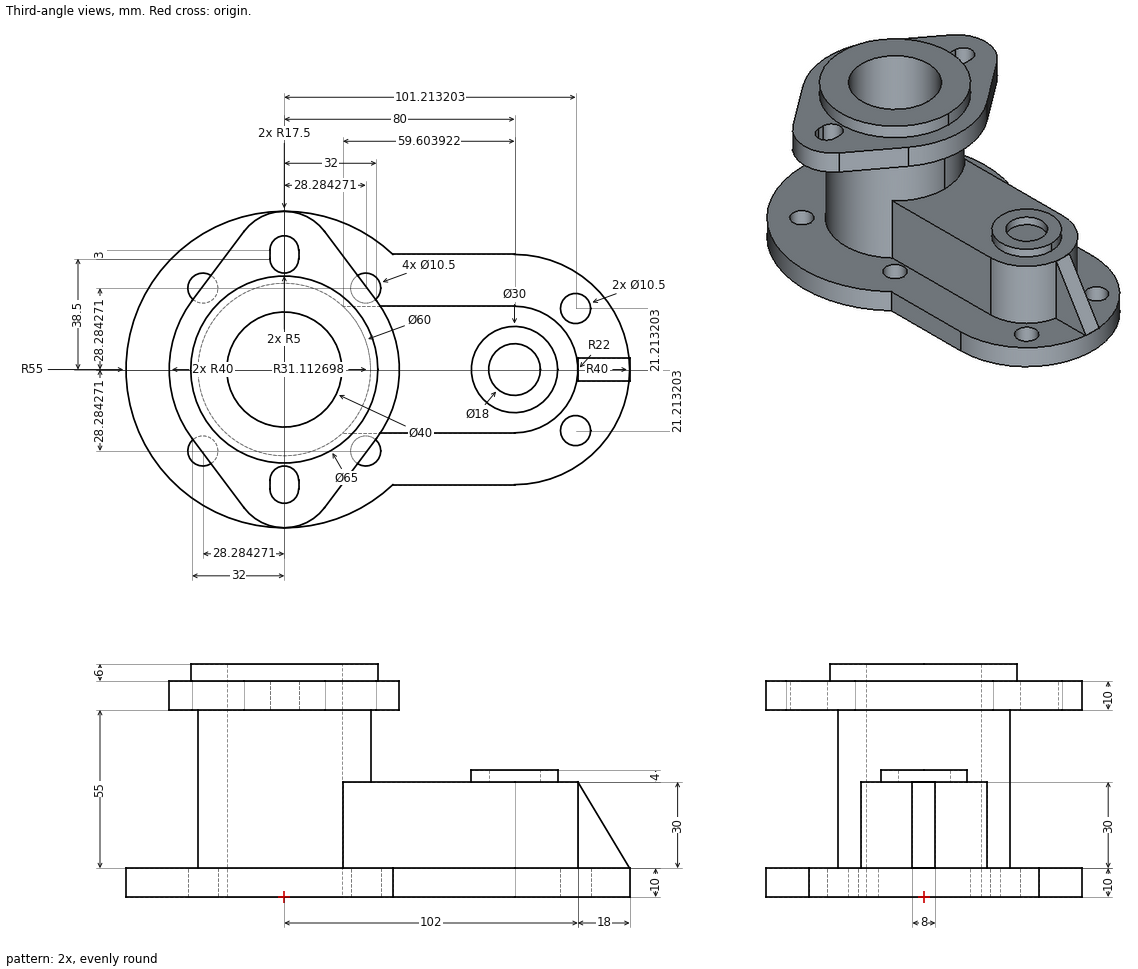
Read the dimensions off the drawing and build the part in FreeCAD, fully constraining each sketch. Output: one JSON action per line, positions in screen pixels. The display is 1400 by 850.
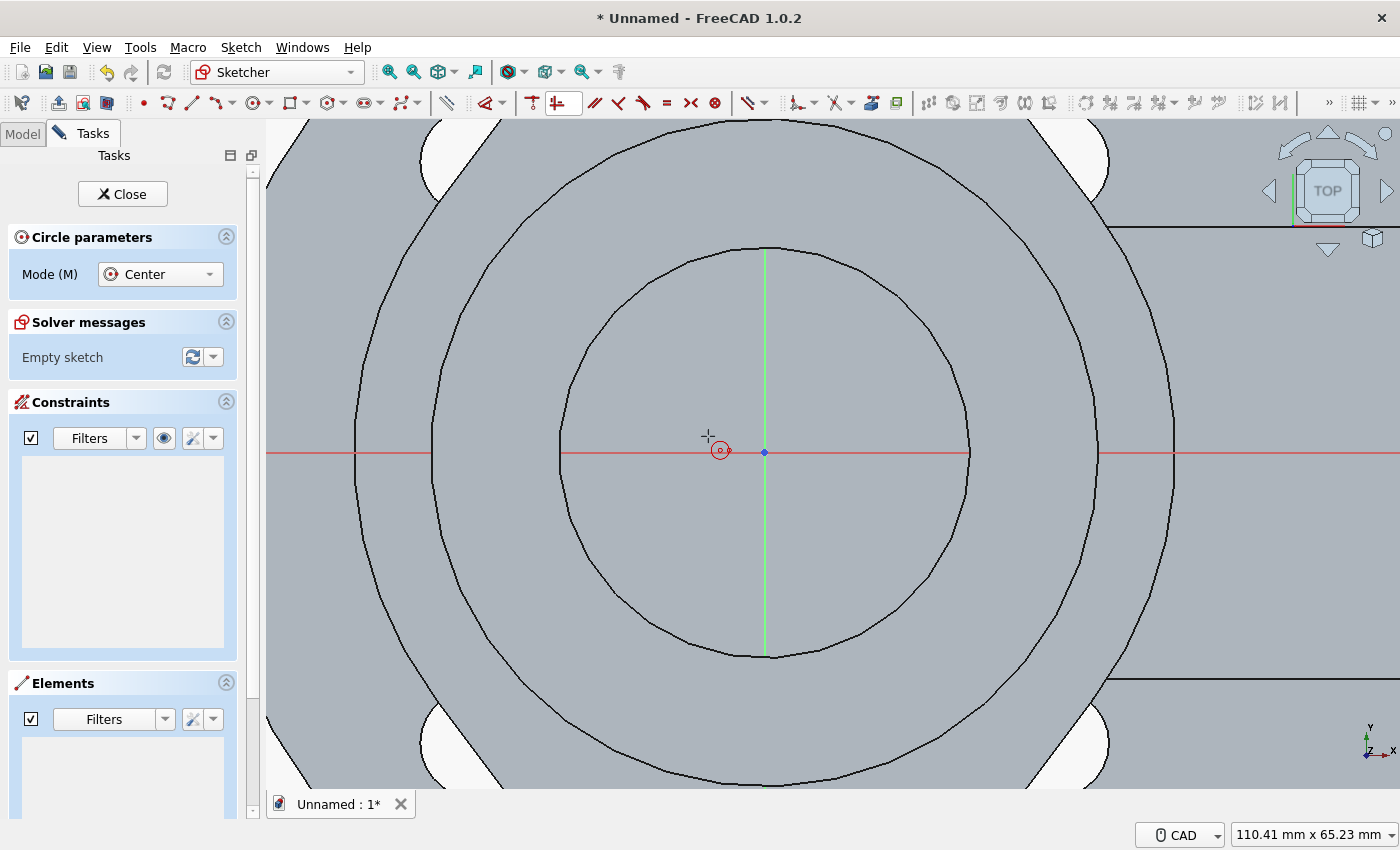
{"action": "left_click", "coordinate": [765, 453]}
{"action": "mouse_move", "coordinate": [910, 307]}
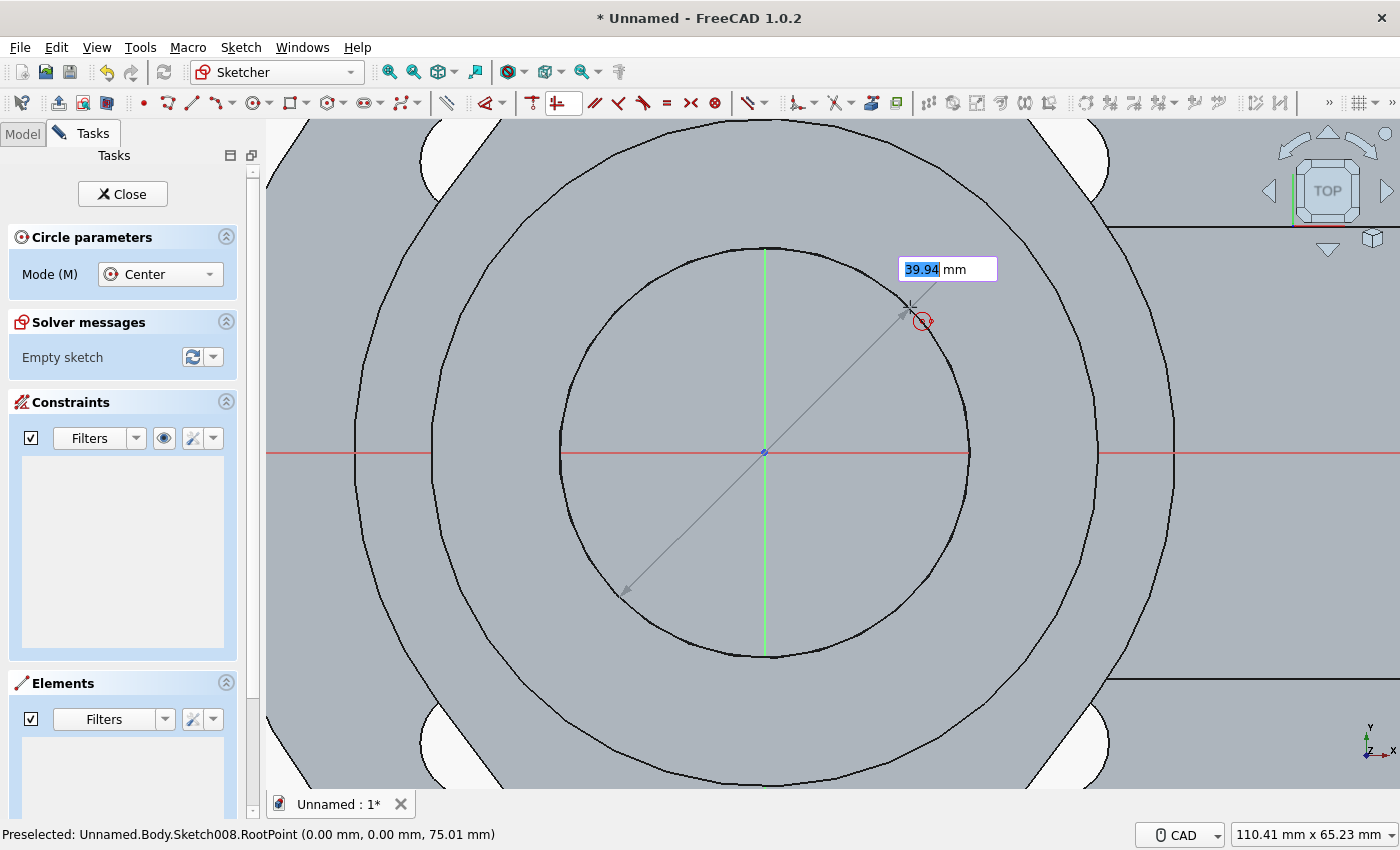
{"action": "type", "text": "40"}
{"action": "key", "text": "Return"}
{"action": "key", "text": "Escape"}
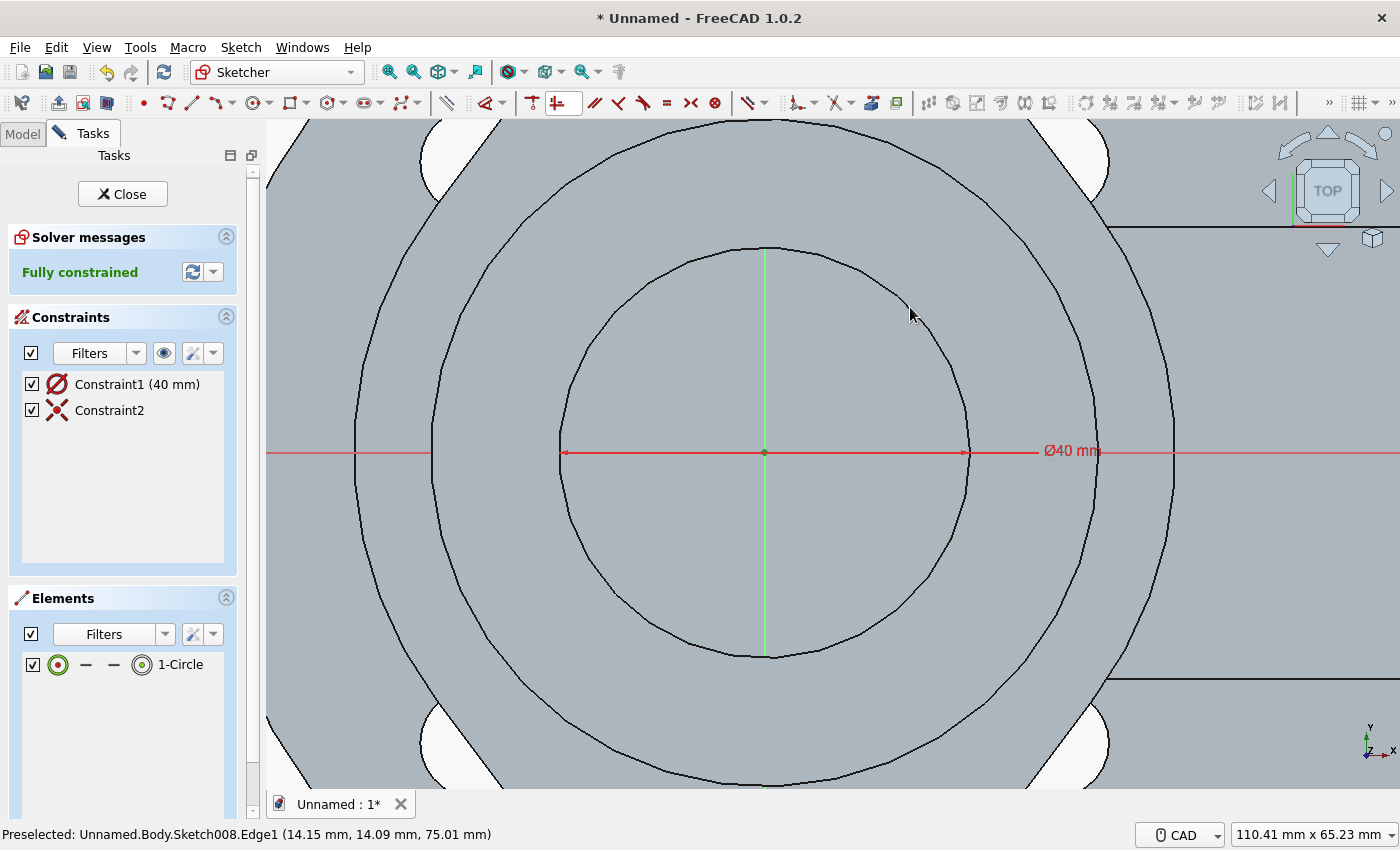
{"action": "left_click", "coordinate": [123, 194]}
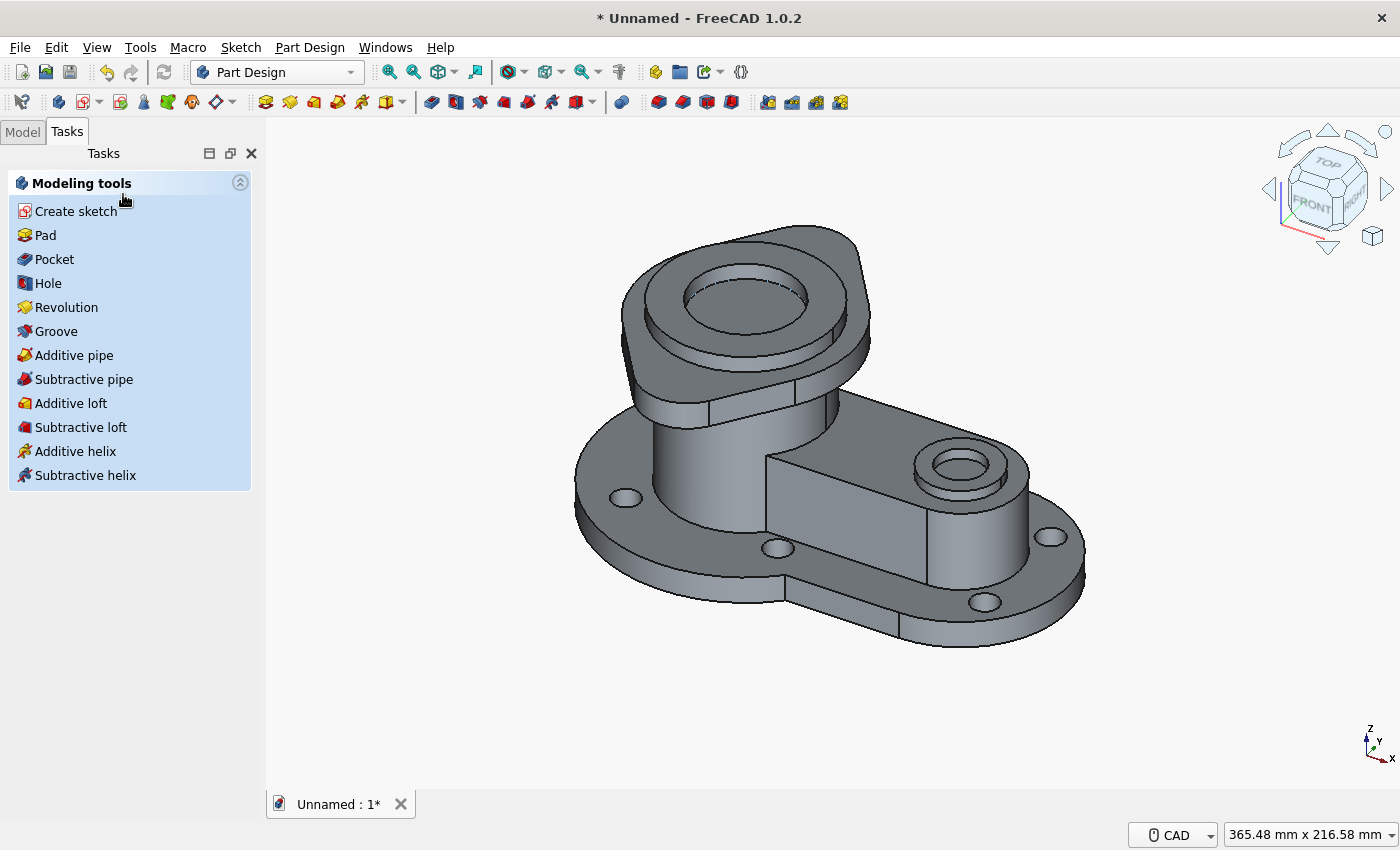
{"action": "left_click", "coordinate": [432, 102]}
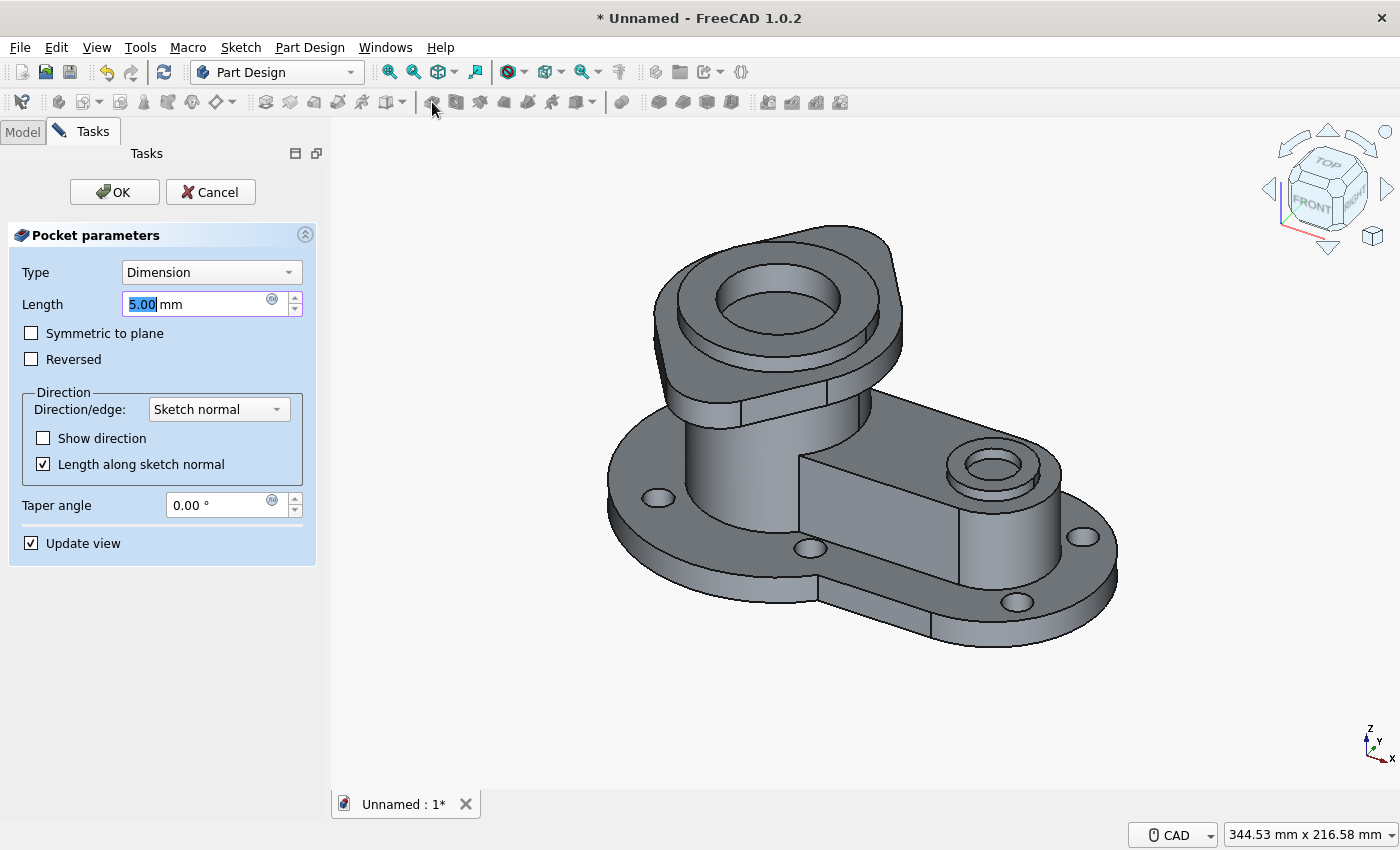
{"action": "left_click", "coordinate": [212, 272]}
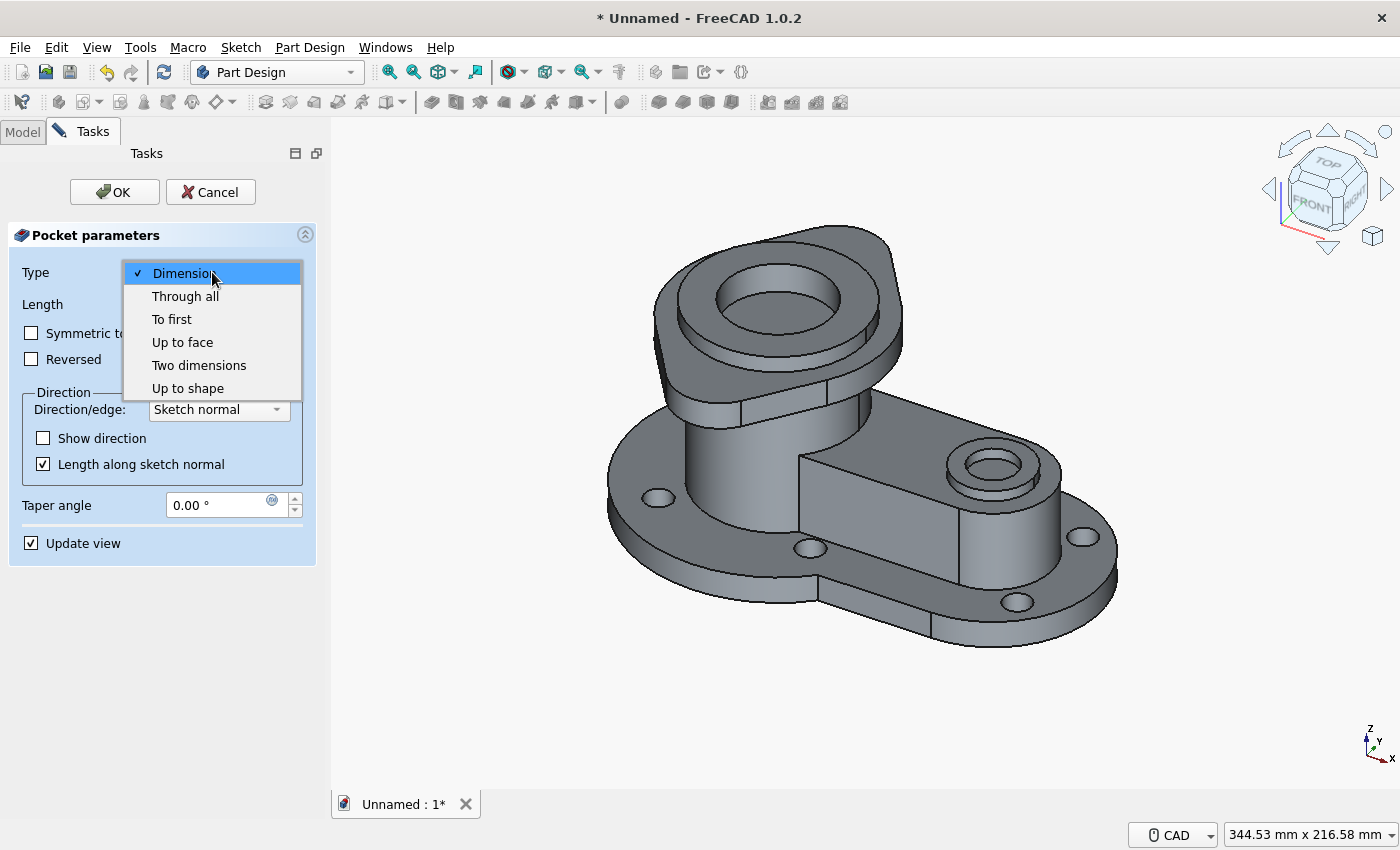
{"action": "left_click", "coordinate": [212, 296]}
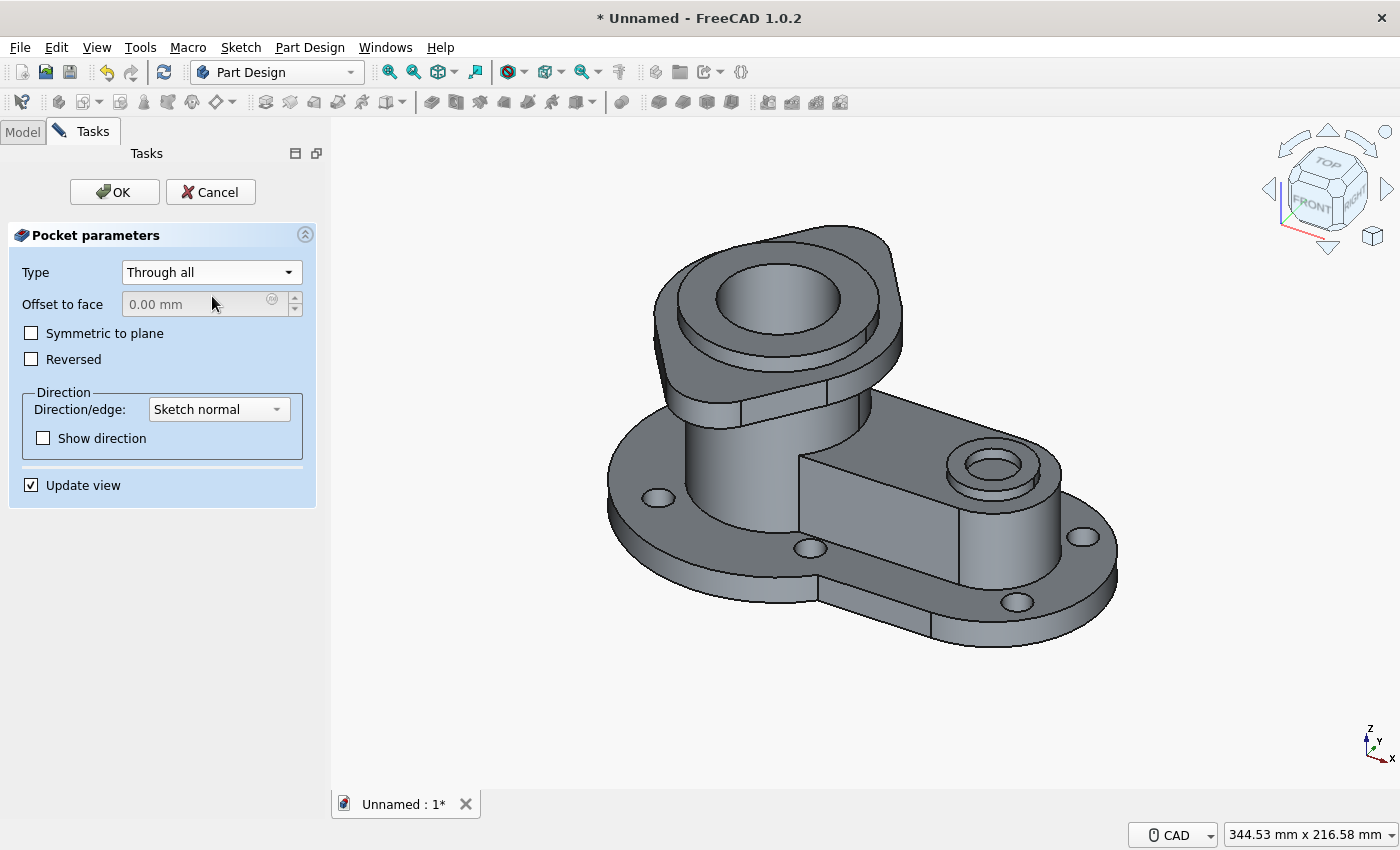
{"action": "left_click", "coordinate": [115, 192]}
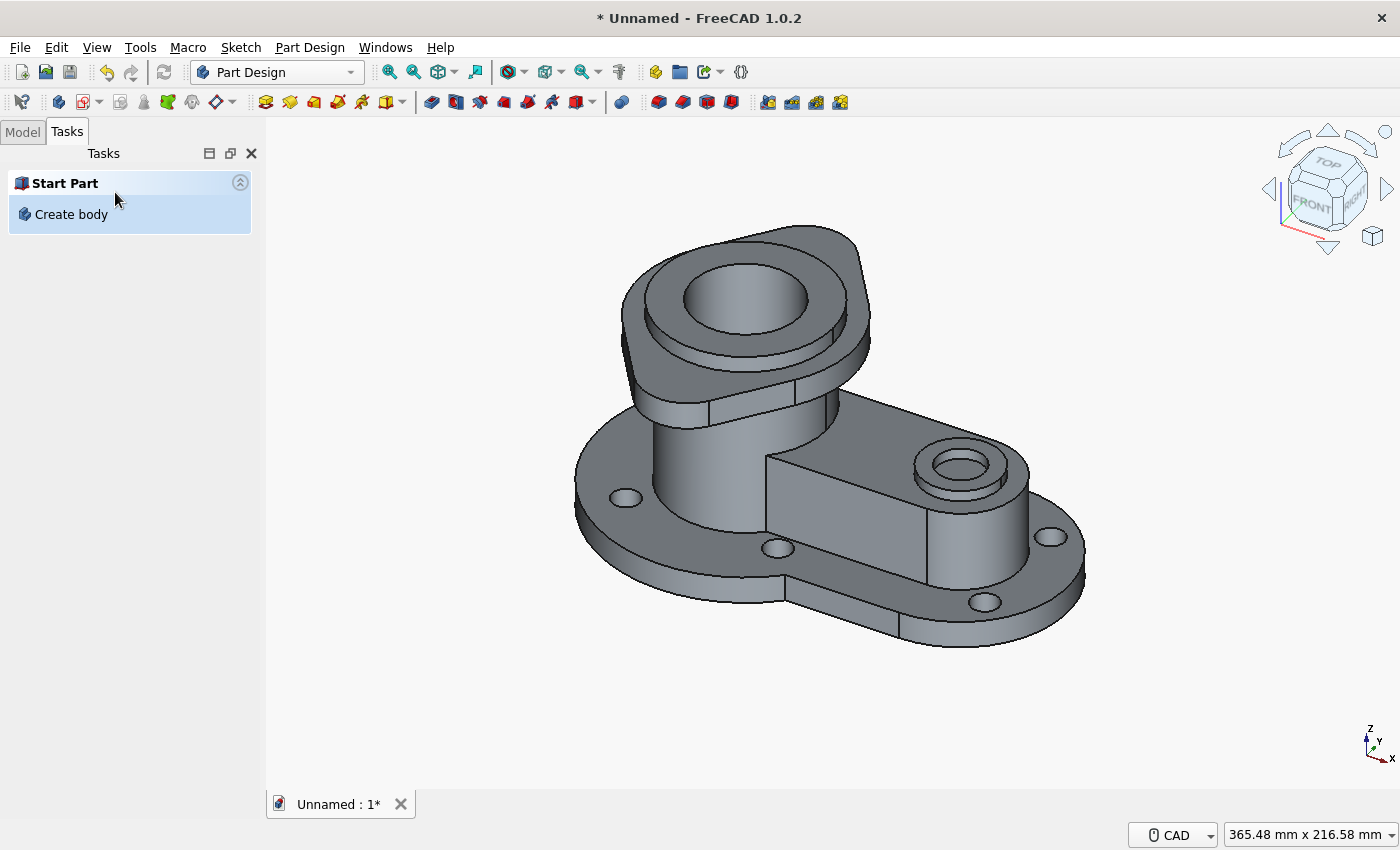
{"action": "left_click", "coordinate": [819, 241]}